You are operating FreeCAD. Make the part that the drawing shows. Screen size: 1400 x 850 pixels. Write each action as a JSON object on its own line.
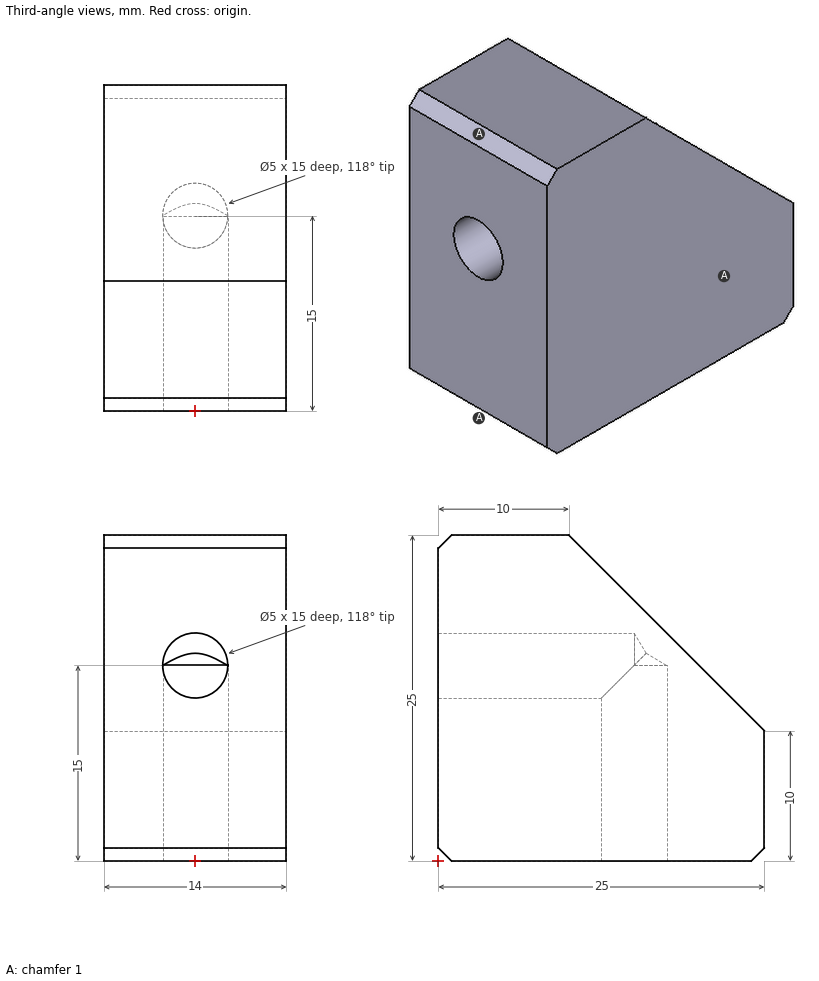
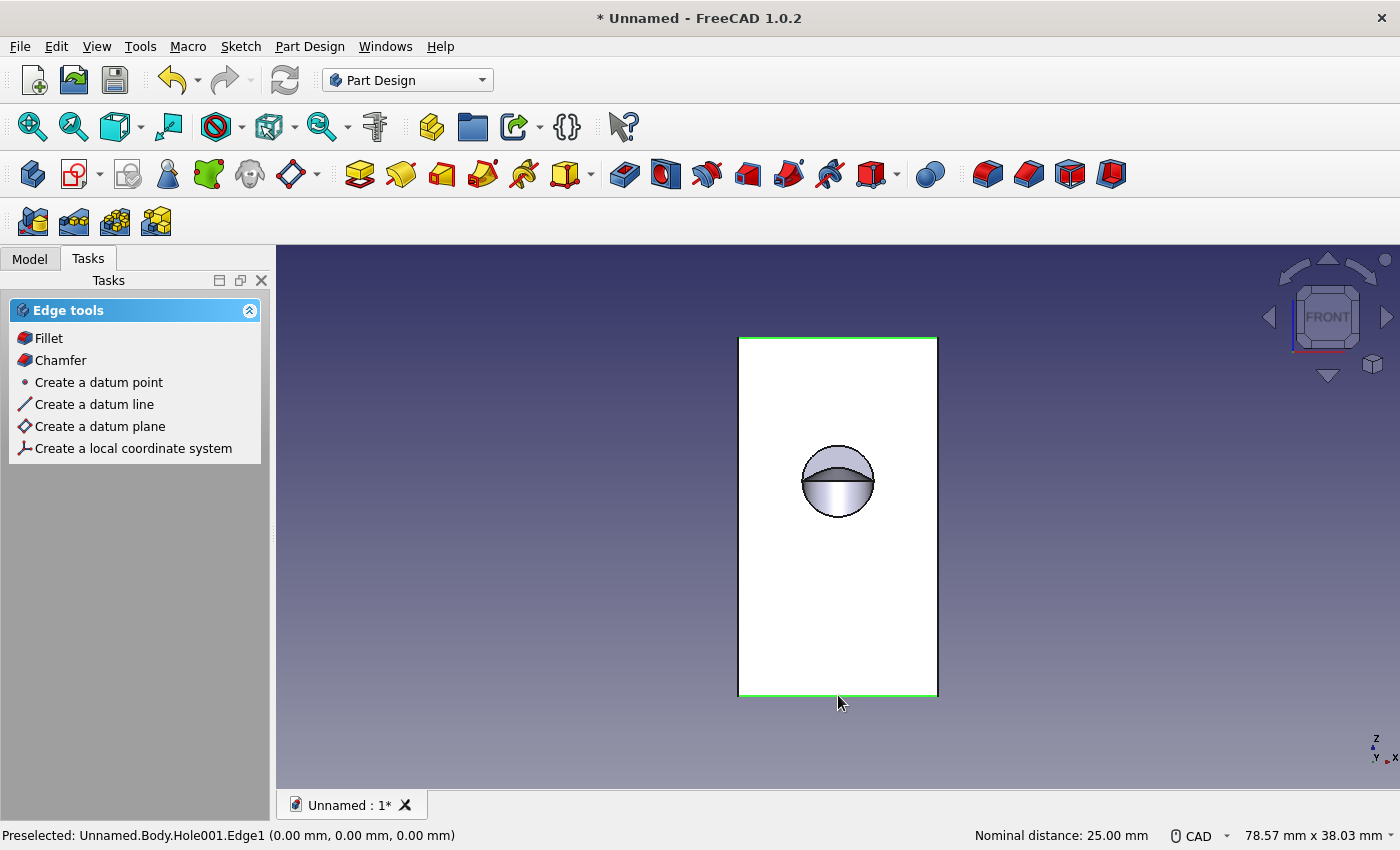
{"action": "key", "text": "3"}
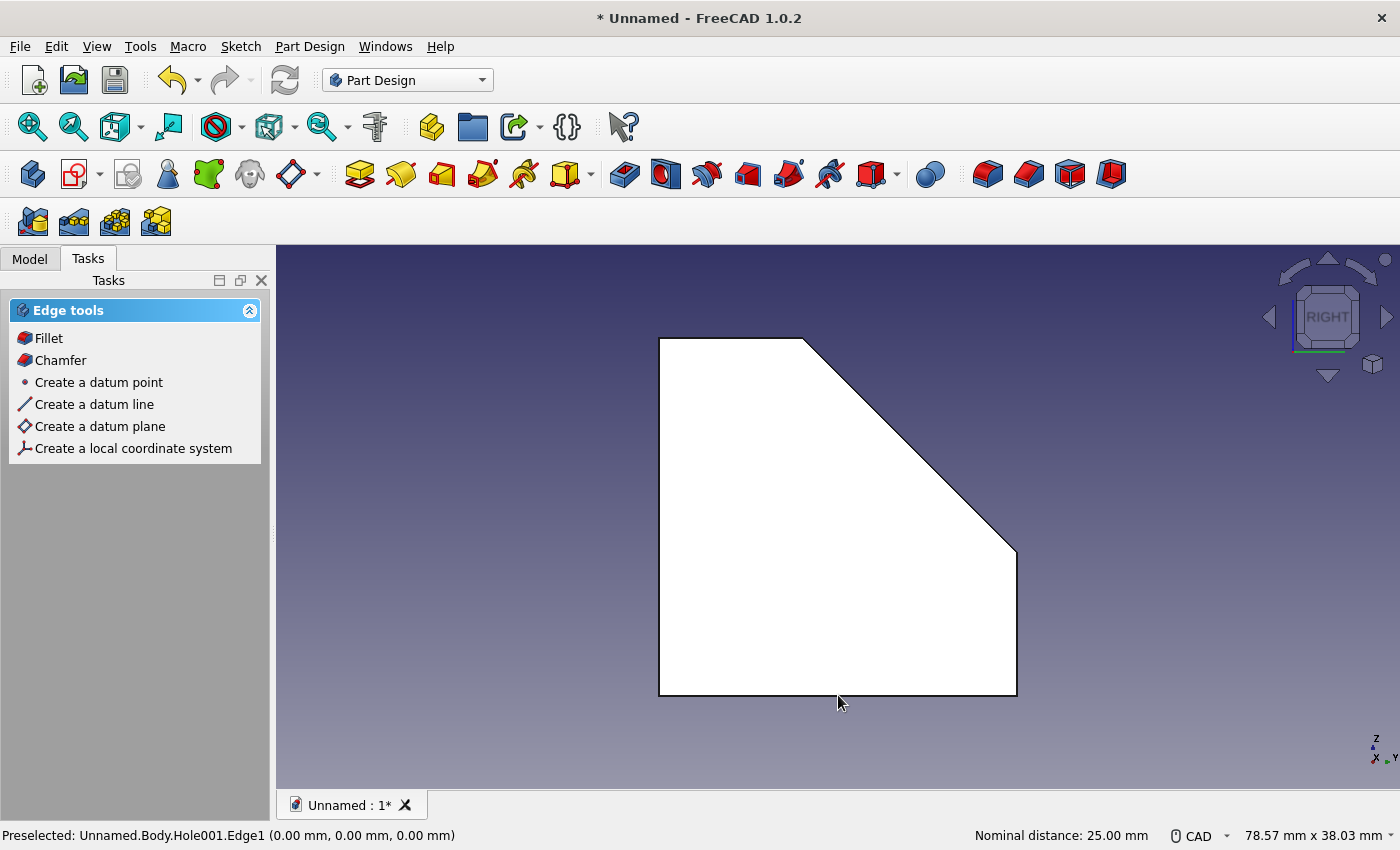
{"action": "key", "text": "5"}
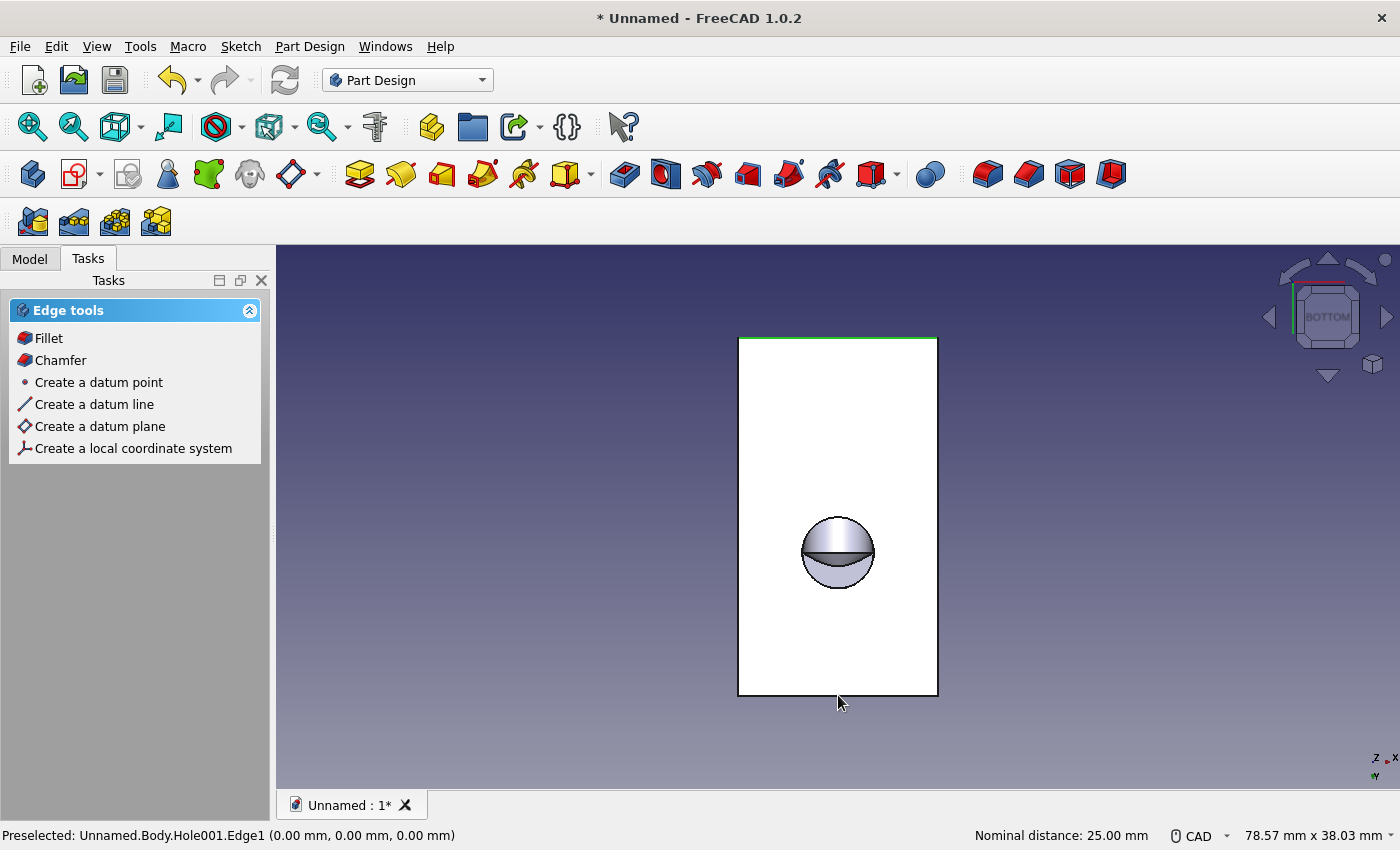
{"action": "left_click", "coordinate": [838, 695], "text": "ctrl"}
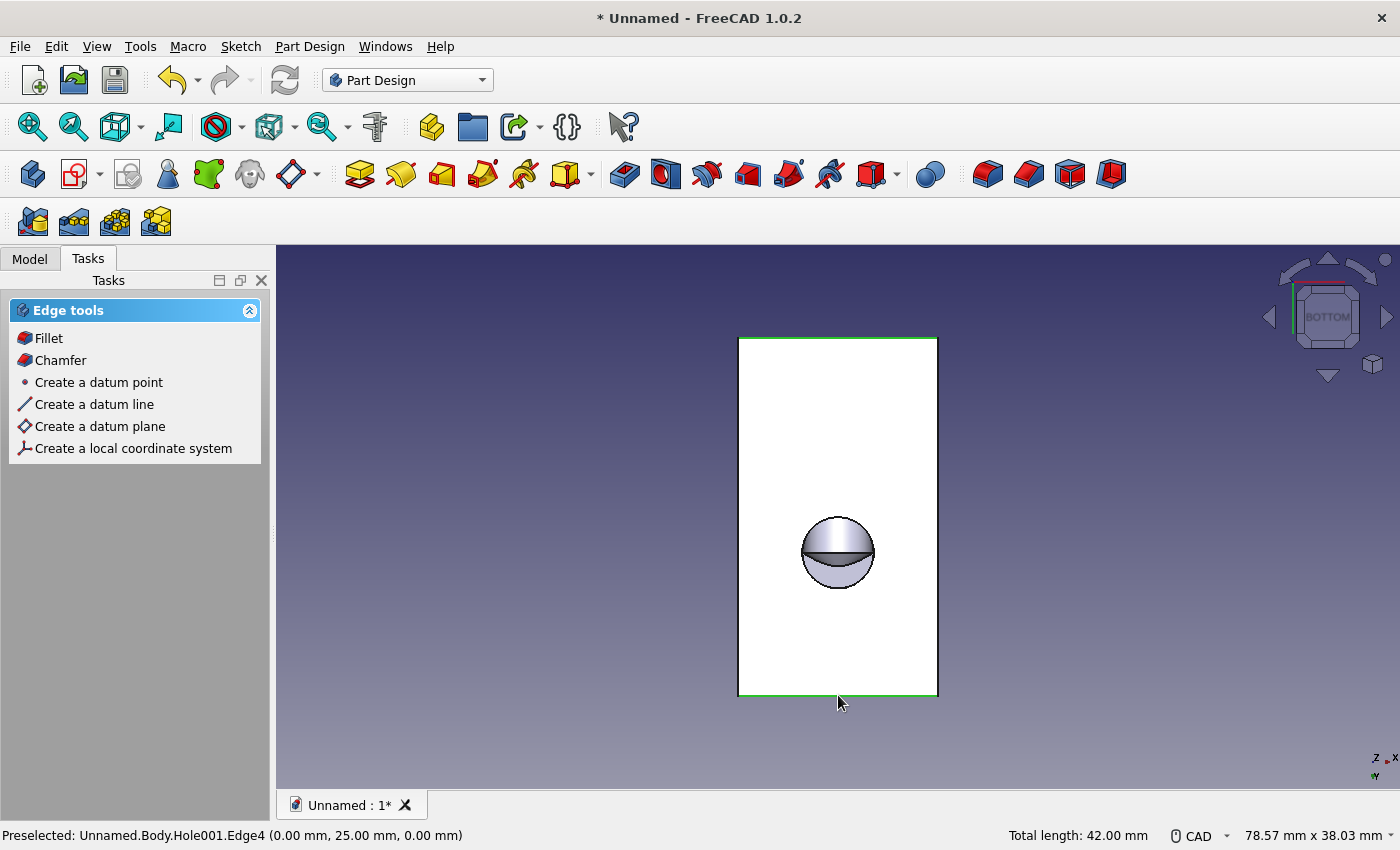
{"action": "left_click", "coordinate": [1029, 174]}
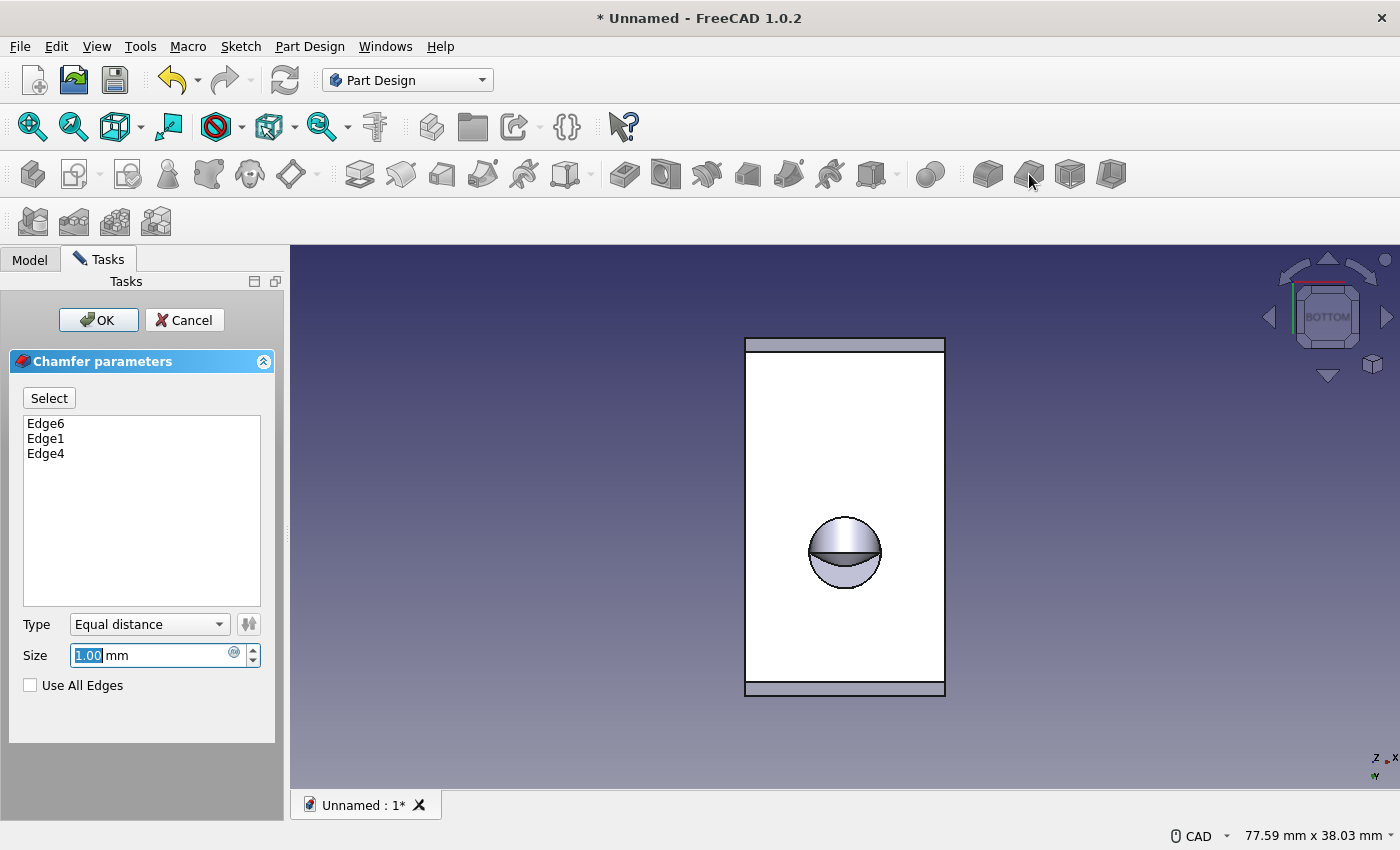
{"action": "type", "text": "1"}
{"action": "key", "text": "Tab"}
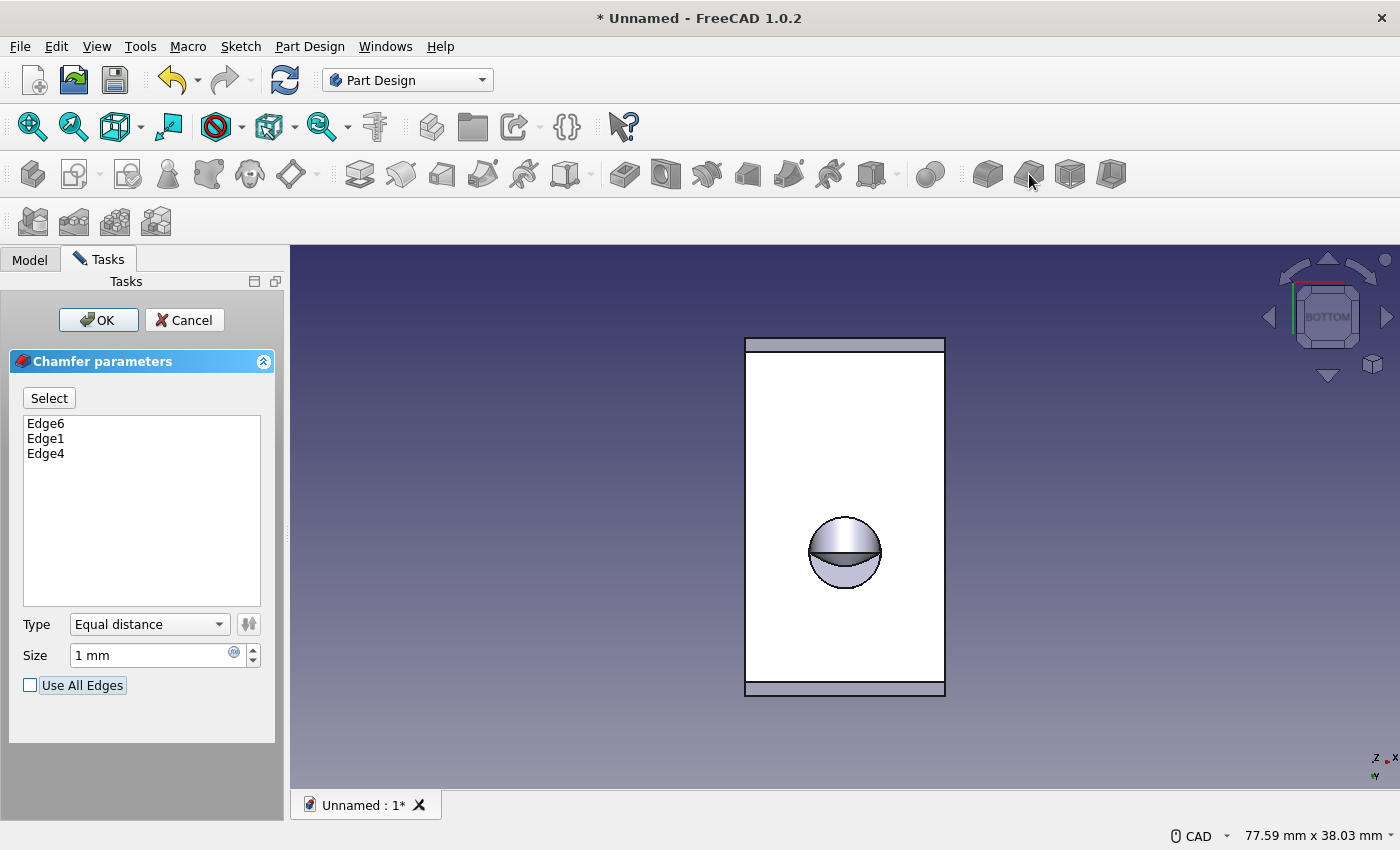
{"action": "left_click", "coordinate": [99, 320]}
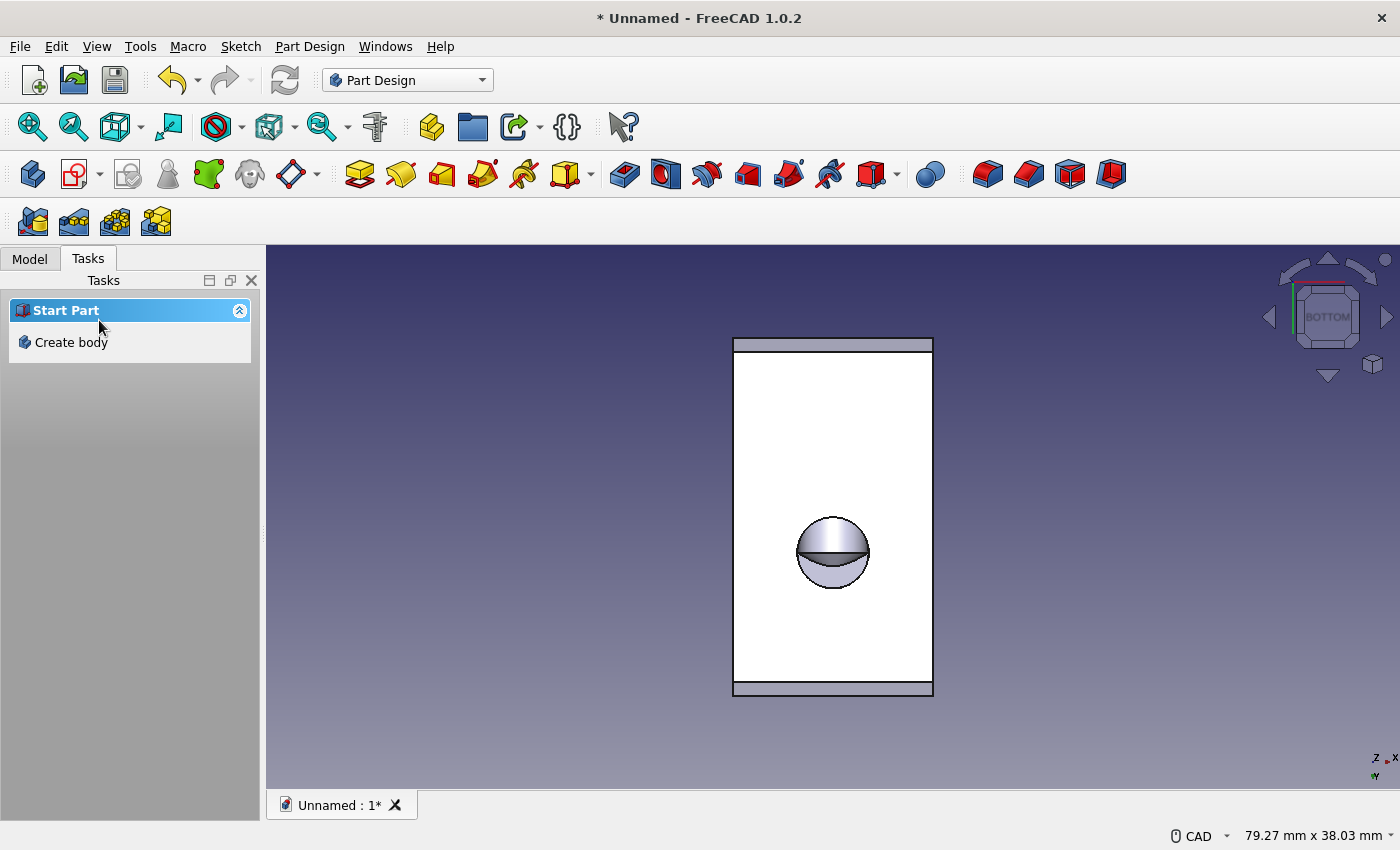
{"action": "key", "text": "0"}